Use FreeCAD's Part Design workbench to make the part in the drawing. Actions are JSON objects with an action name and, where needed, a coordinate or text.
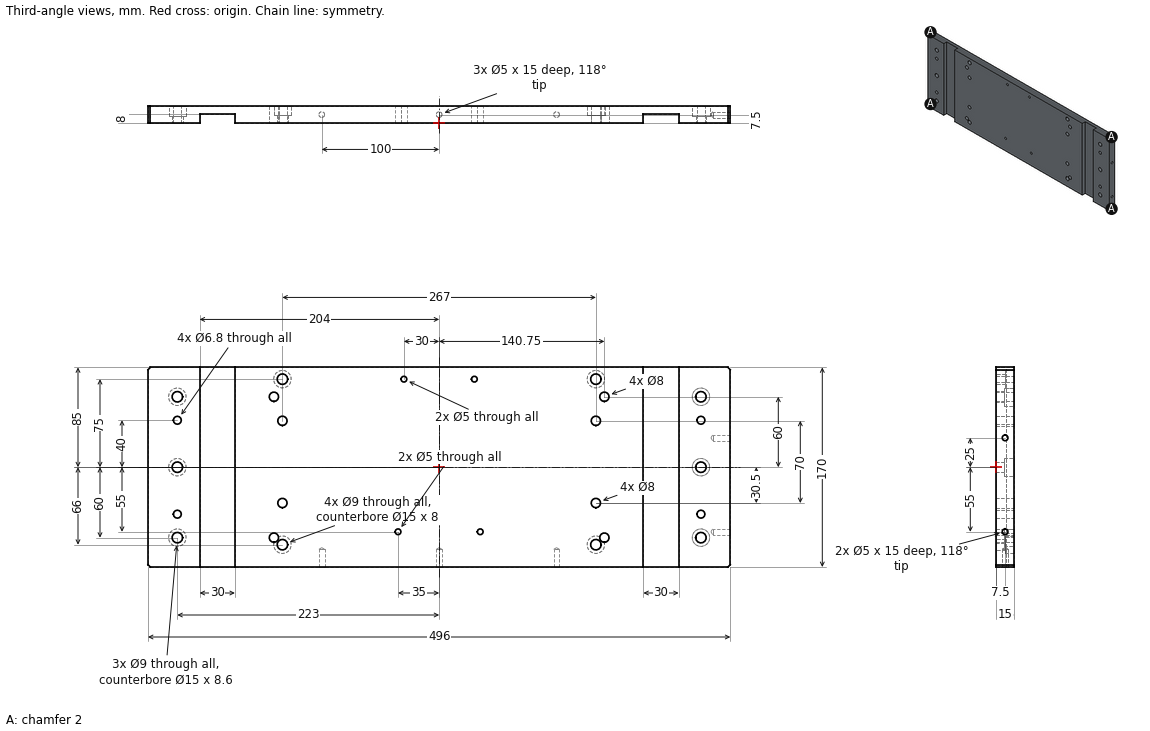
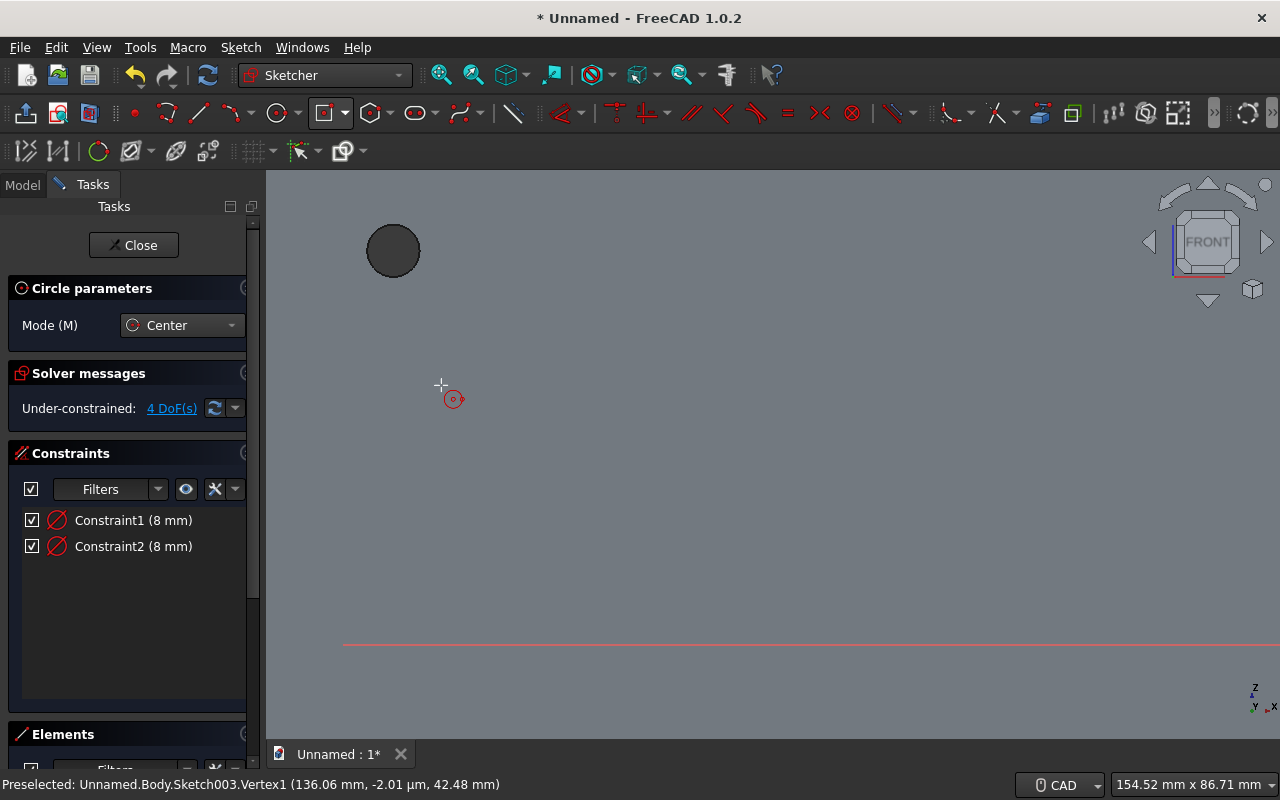
{"action": "left_click", "coordinate": [441, 385]}
{"action": "mouse_move", "coordinate": [460, 367]}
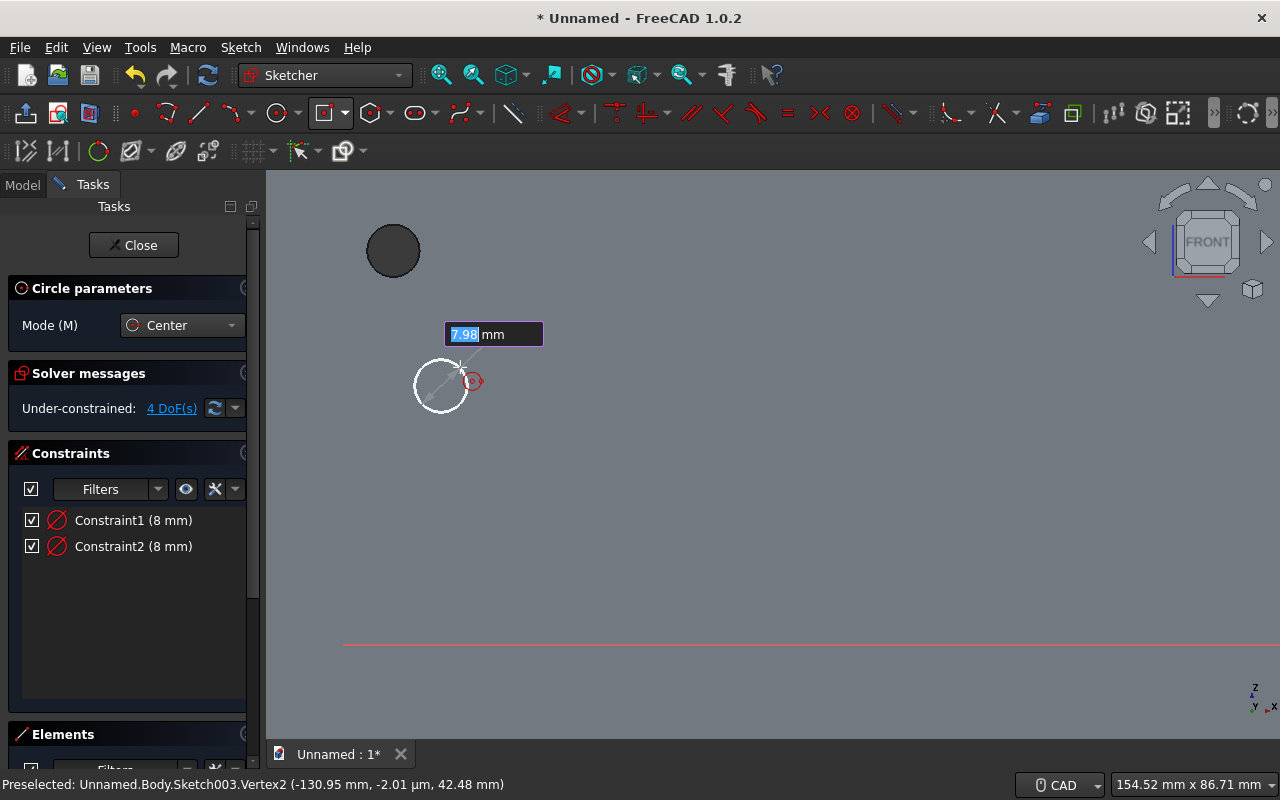
{"action": "type", "text": "8"}
{"action": "key", "text": "Return"}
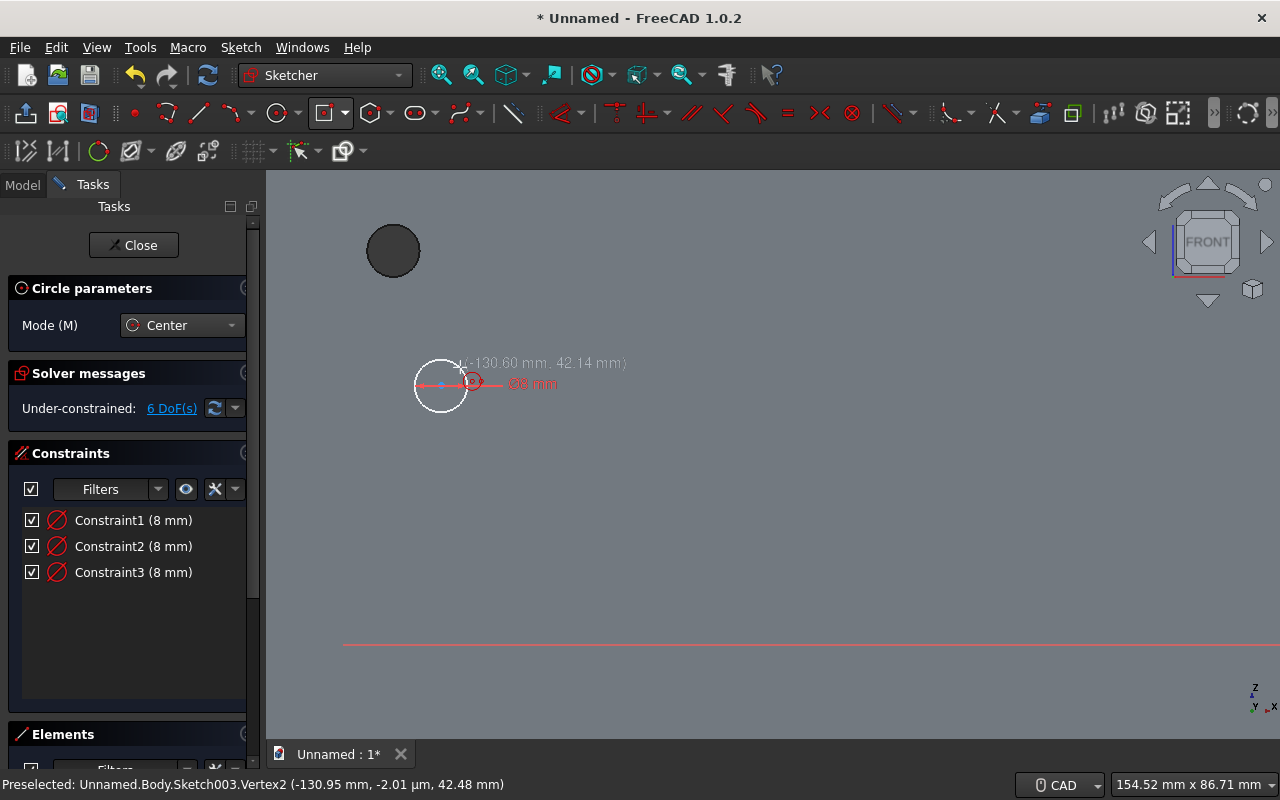
{"action": "scroll", "coordinate": [440, 385], "scroll_direction": "down", "scroll_amount": 6}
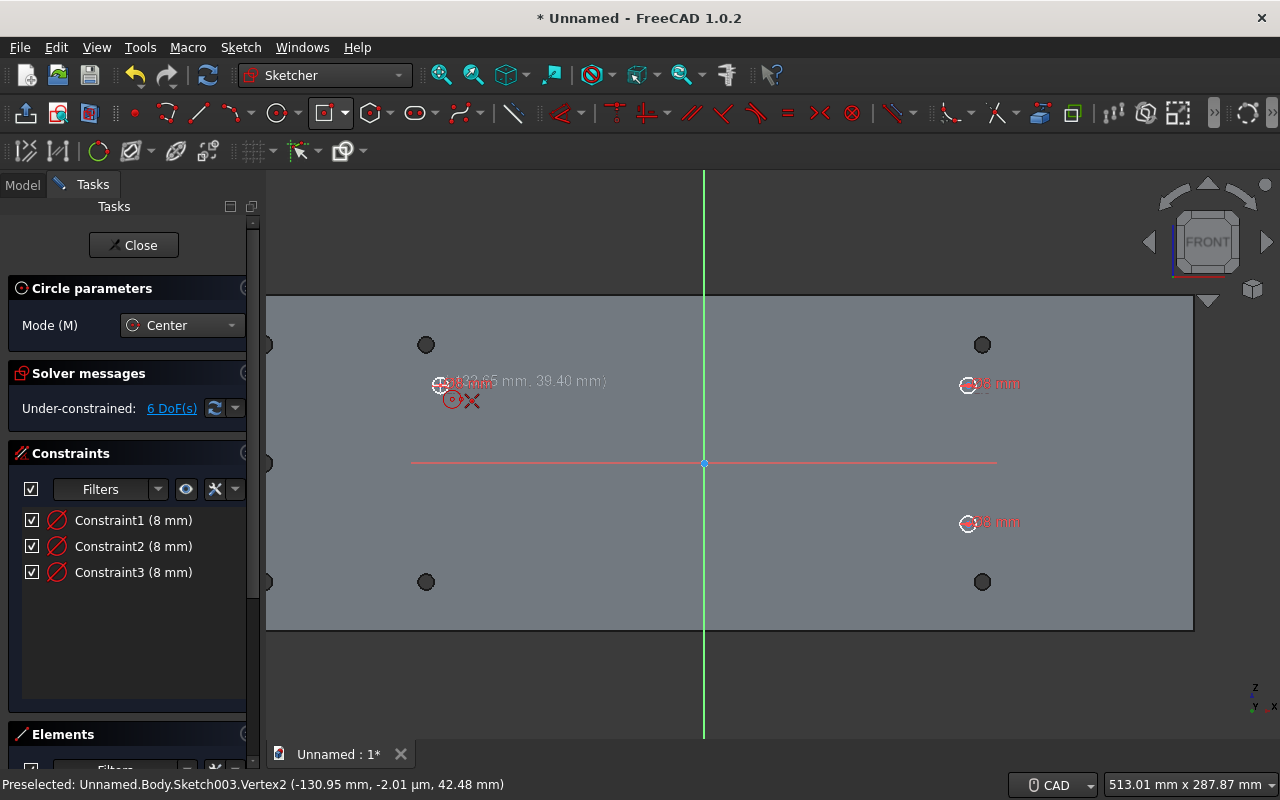
{"action": "scroll", "coordinate": [440, 524], "scroll_direction": "up", "scroll_amount": 6}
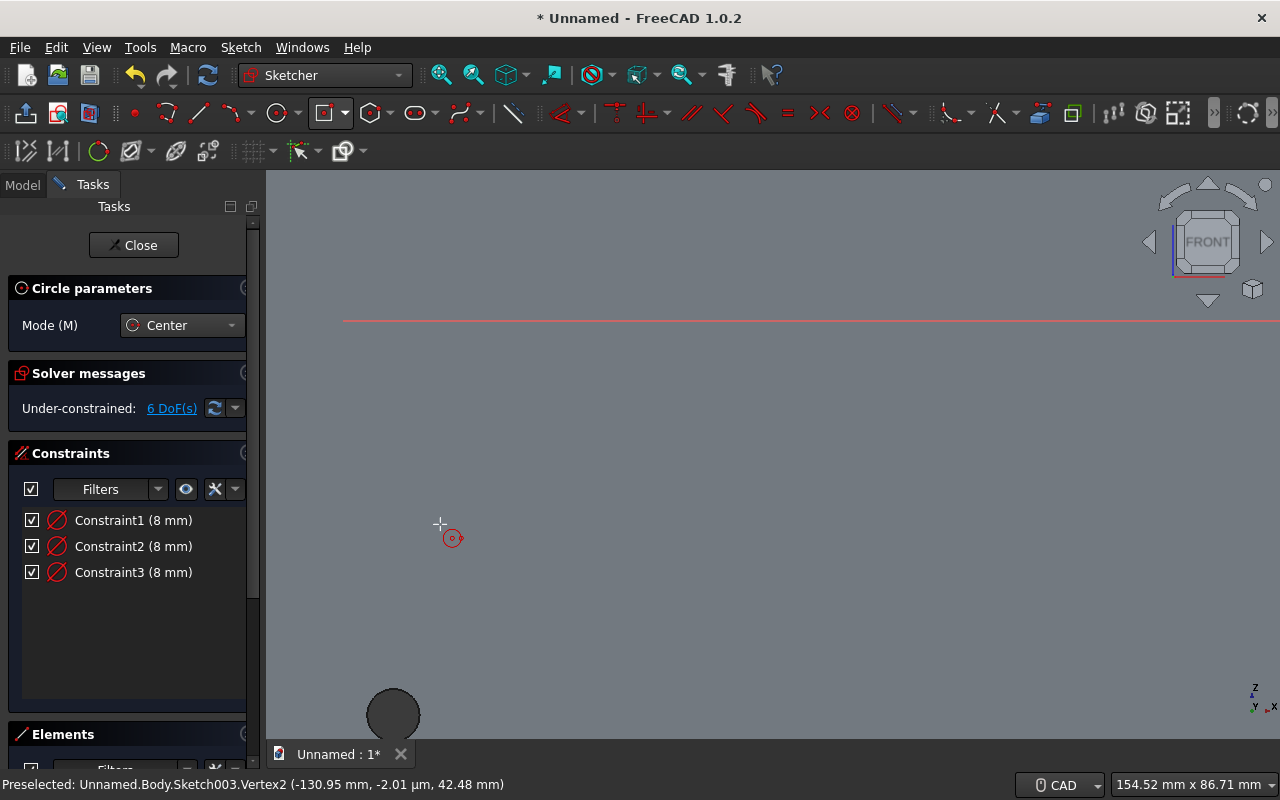
{"action": "left_click", "coordinate": [441, 522]}
{"action": "mouse_move", "coordinate": [460, 503]}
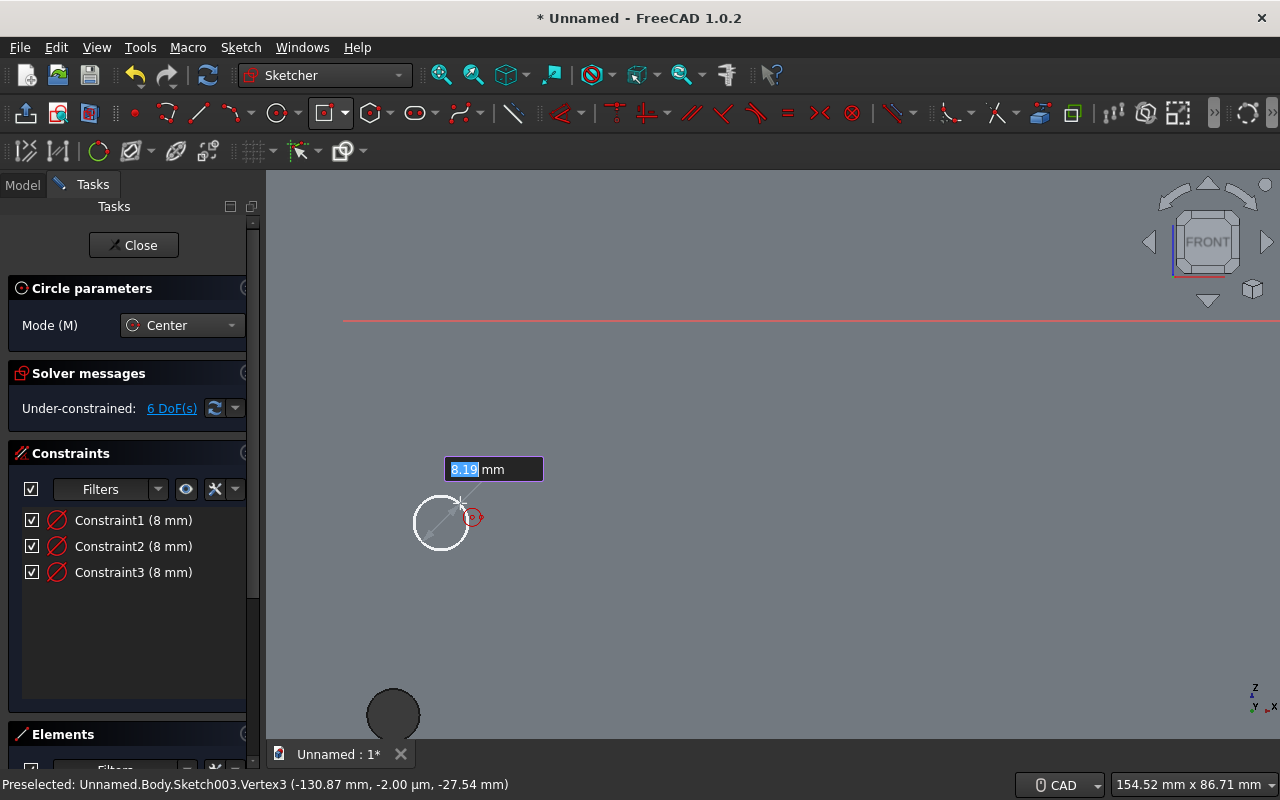
{"action": "type", "text": "8"}
{"action": "key", "text": "Return"}
{"action": "key", "text": "Escape"}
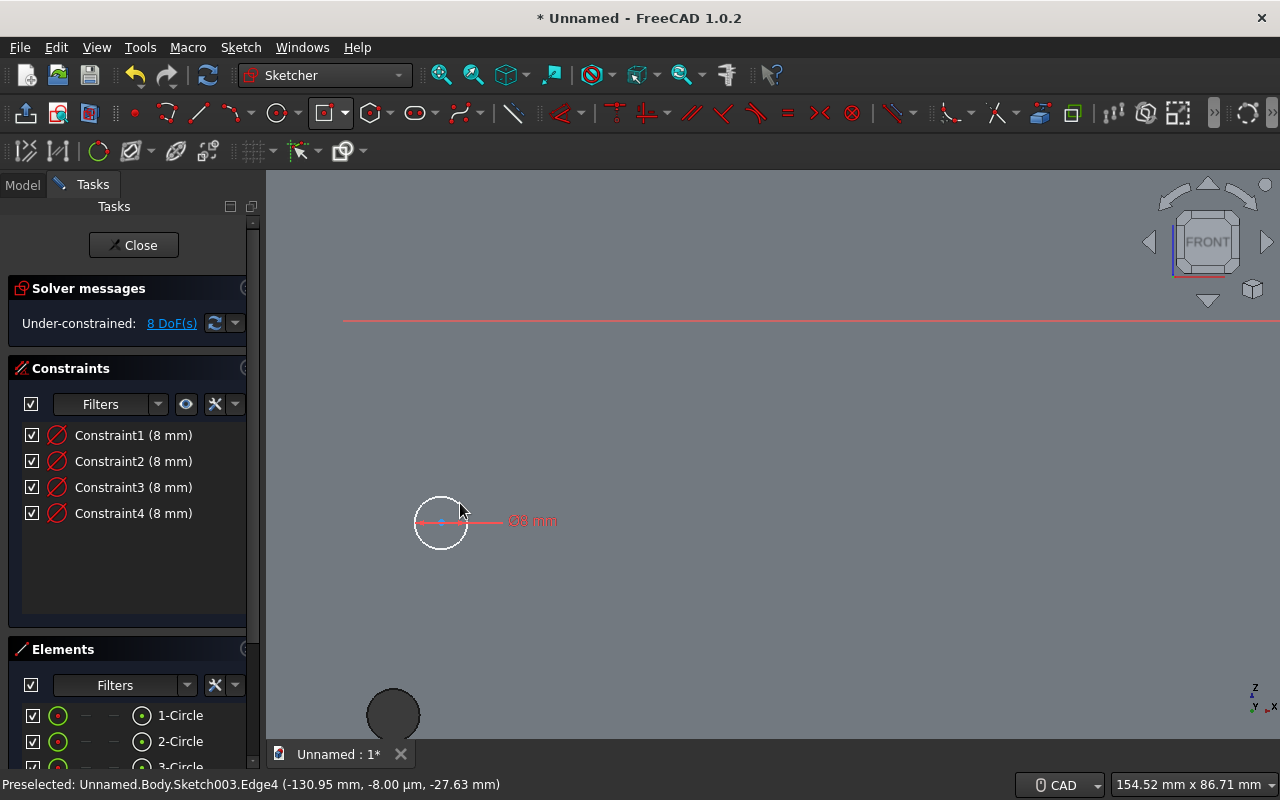
{"action": "scroll", "coordinate": [440, 525], "scroll_direction": "down", "scroll_amount": 6}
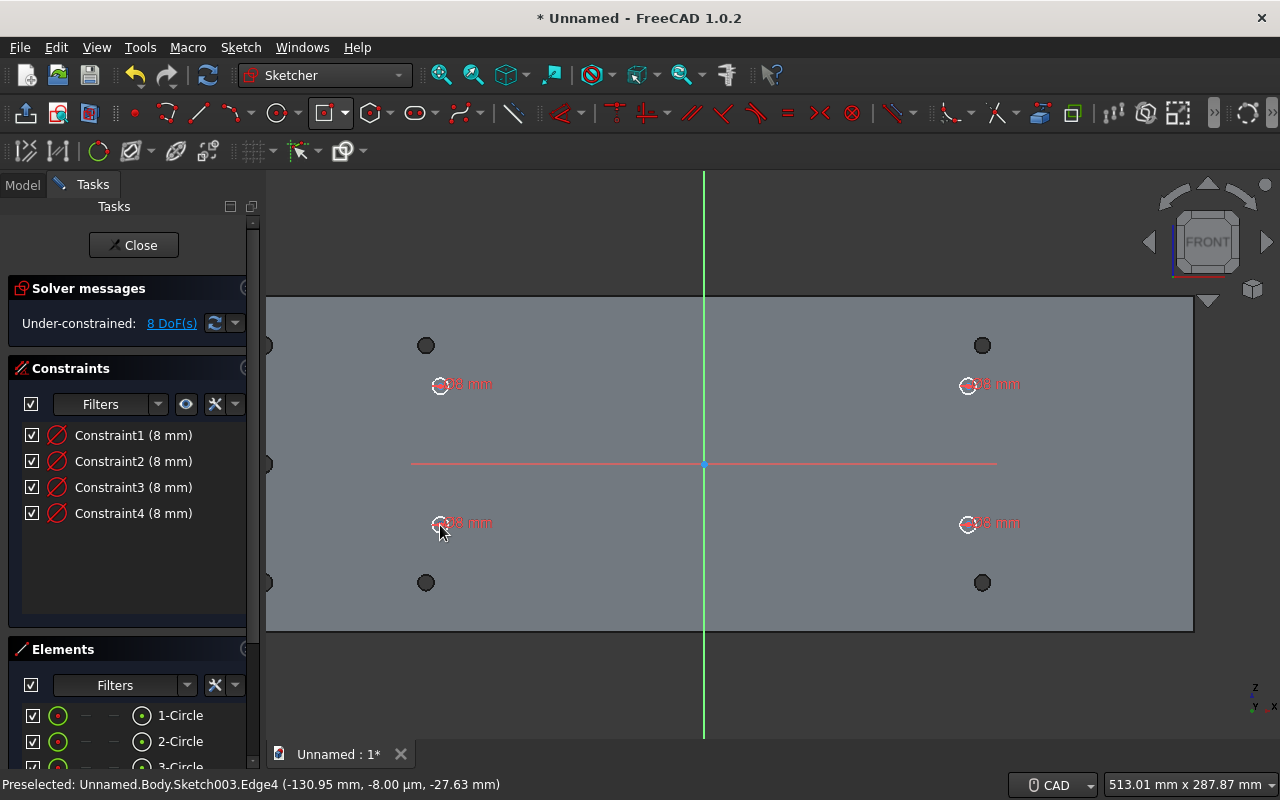
{"action": "left_click", "coordinate": [968, 386]}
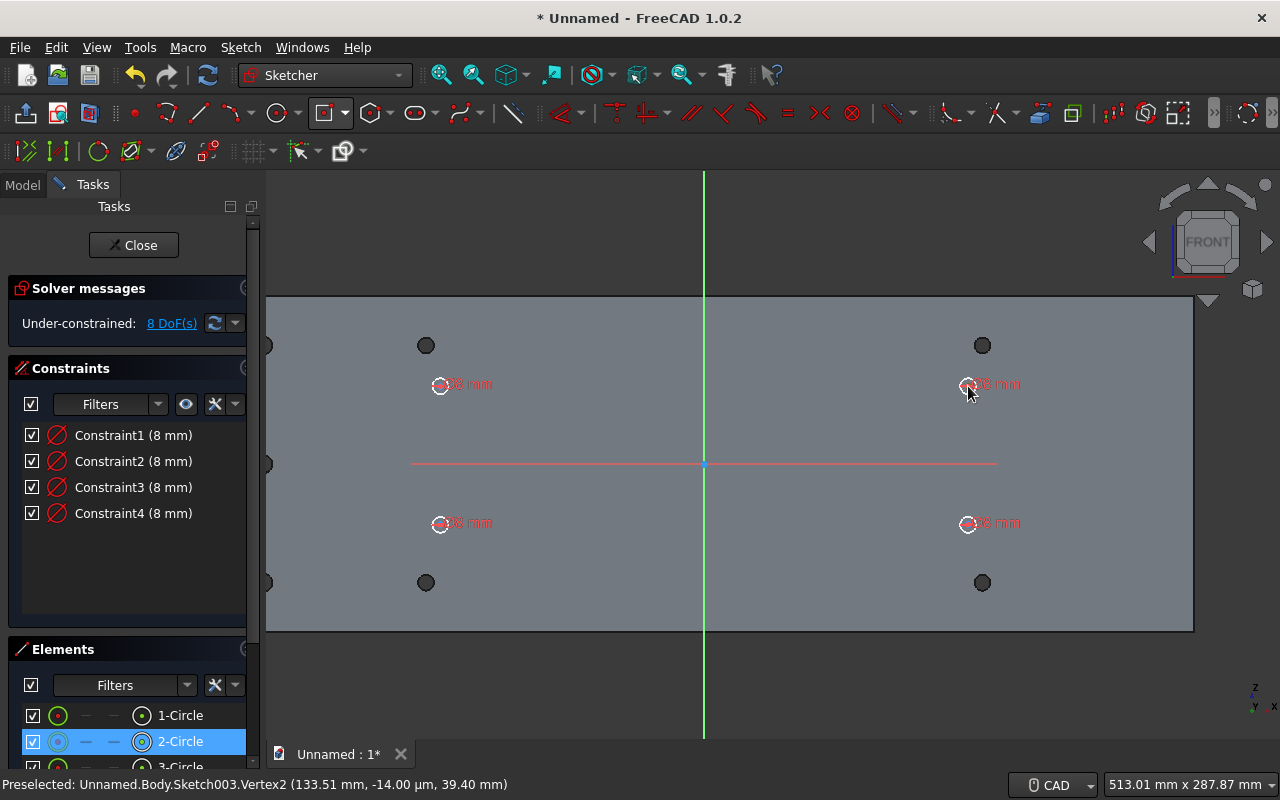
{"action": "left_click", "coordinate": [440, 386]}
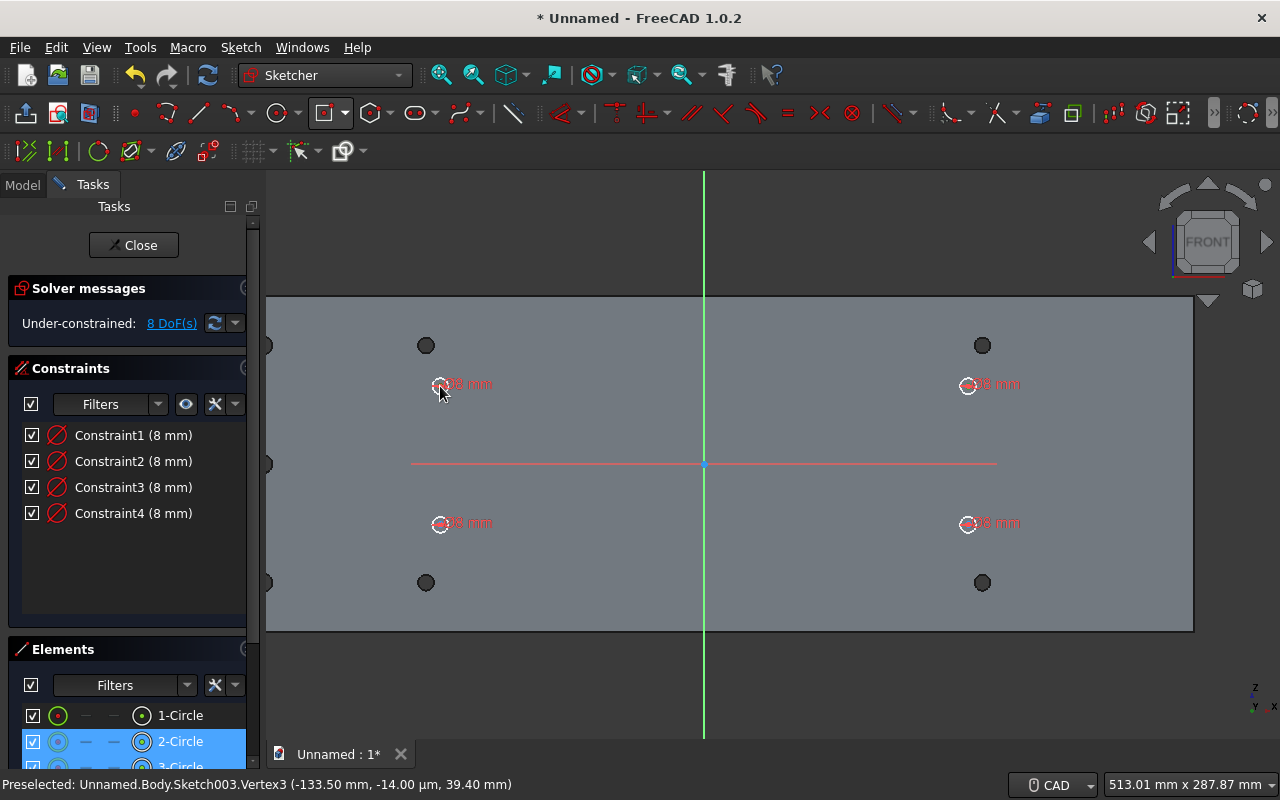
{"action": "left_click", "coordinate": [704, 674]}